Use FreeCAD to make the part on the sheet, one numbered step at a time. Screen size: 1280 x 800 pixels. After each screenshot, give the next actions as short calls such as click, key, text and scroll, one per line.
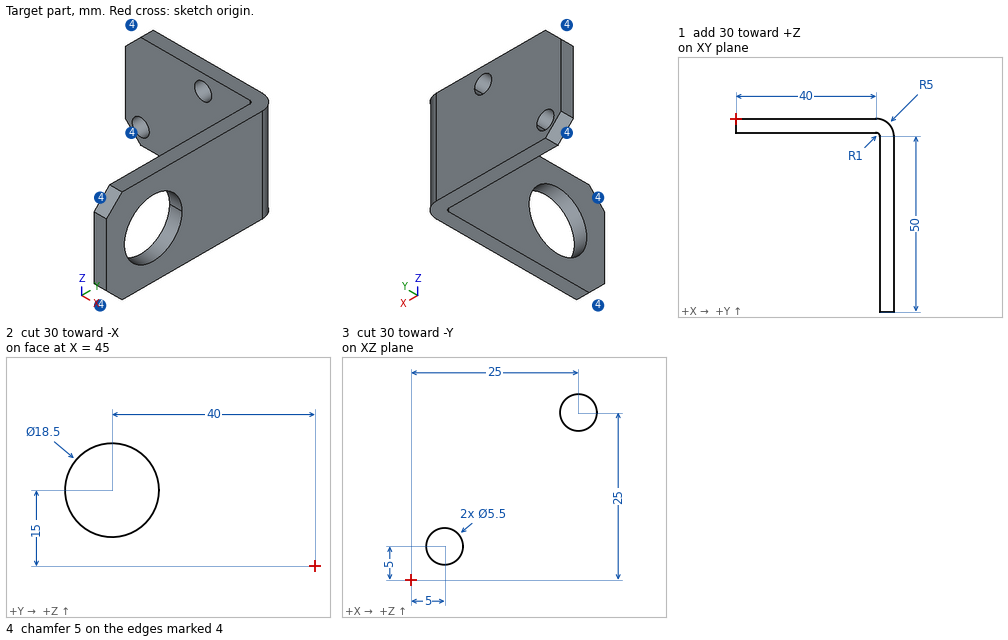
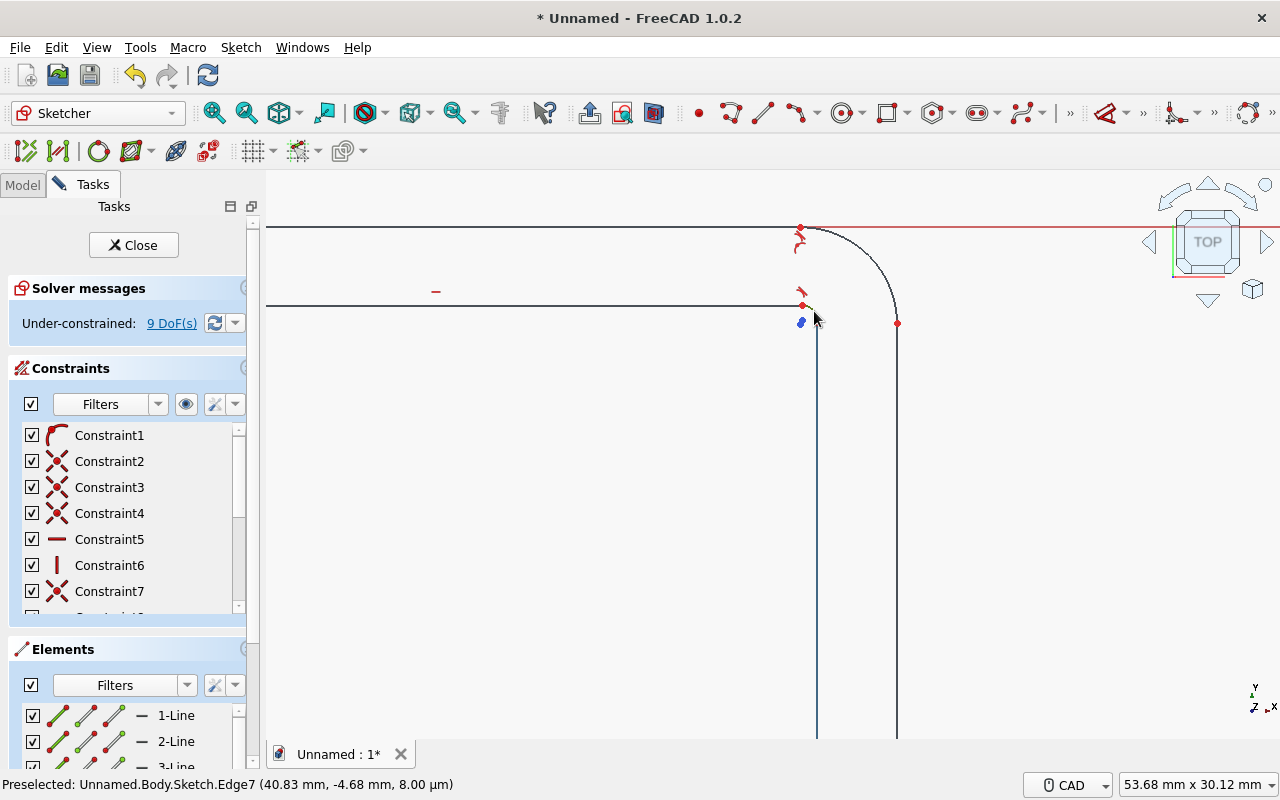
key(t)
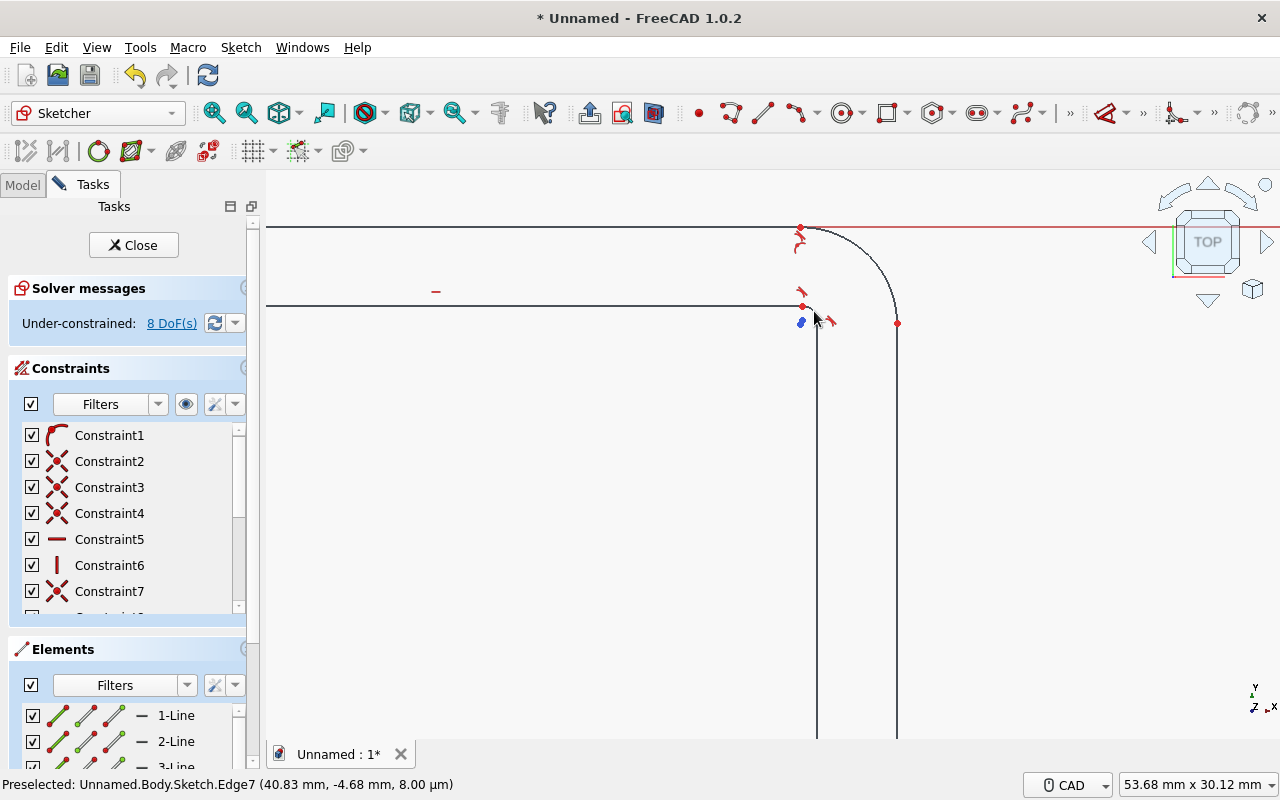
click(897, 608)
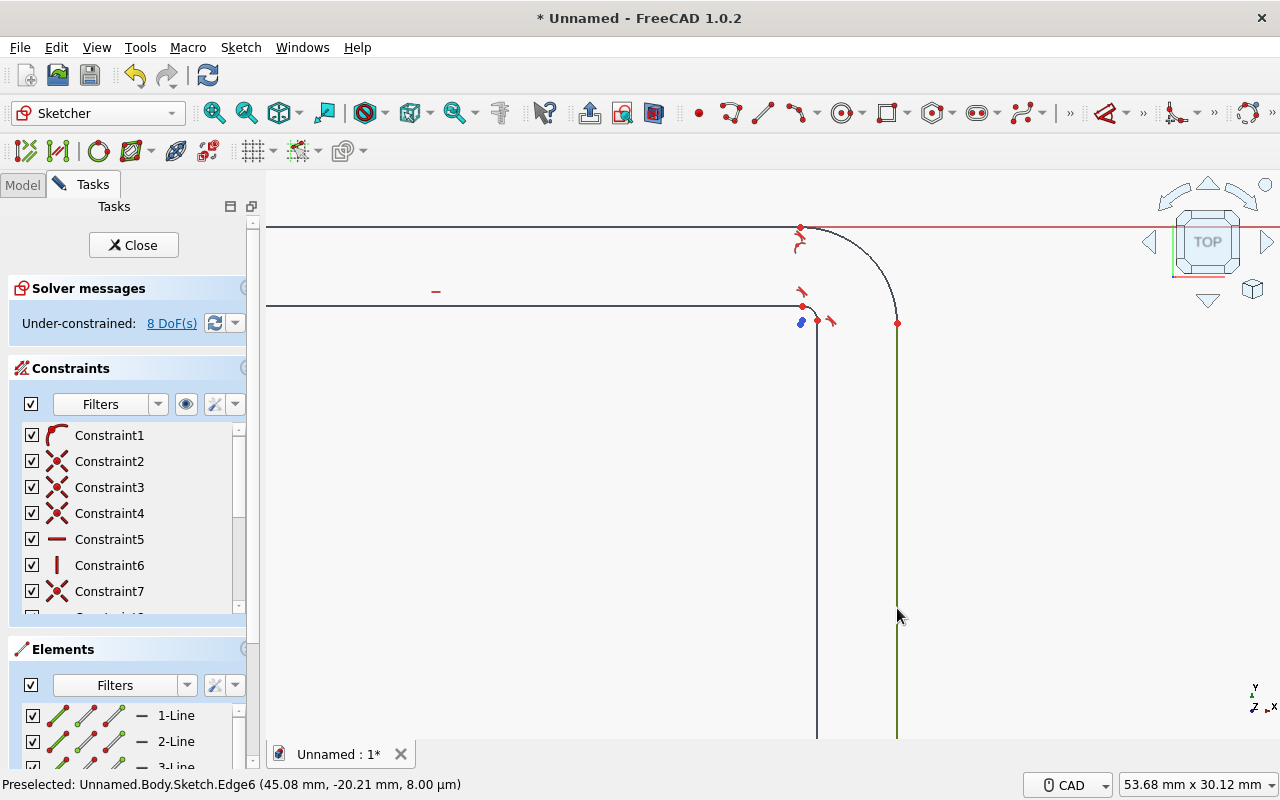
click(886, 280)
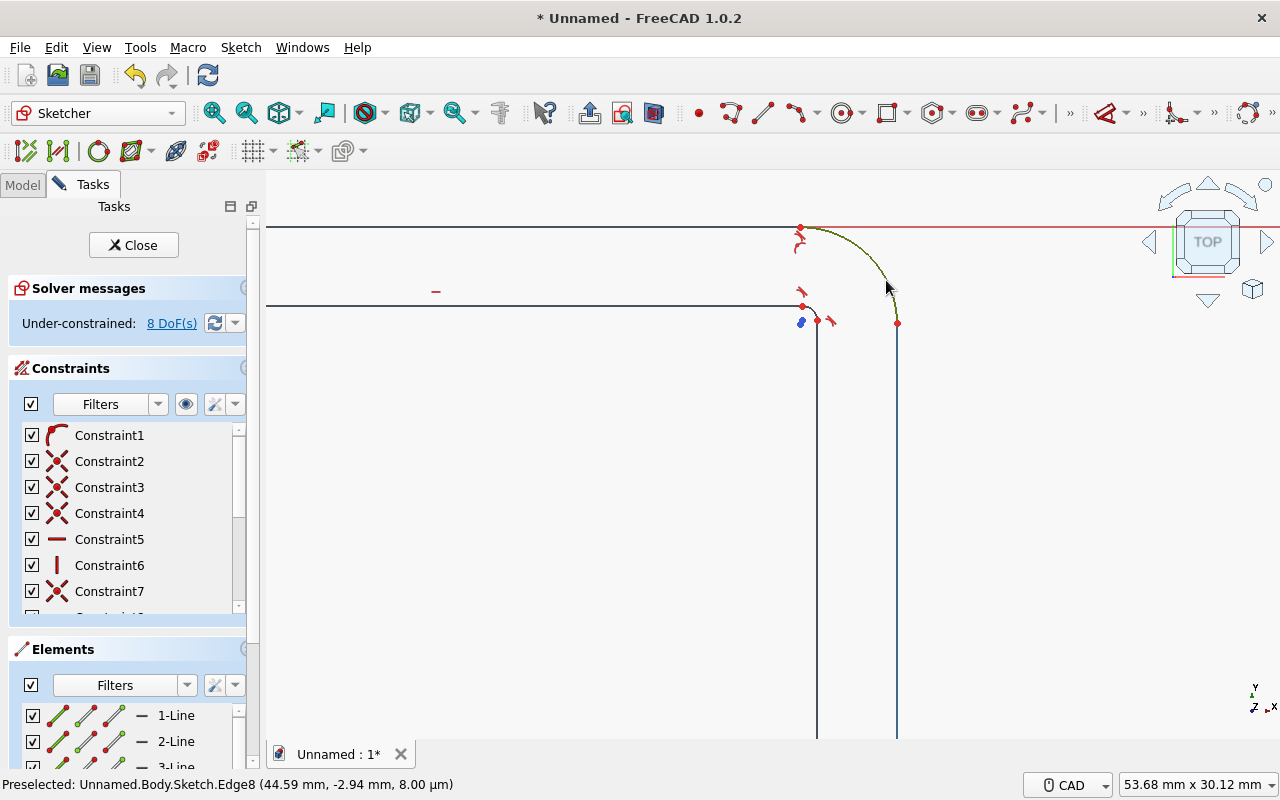
key(t)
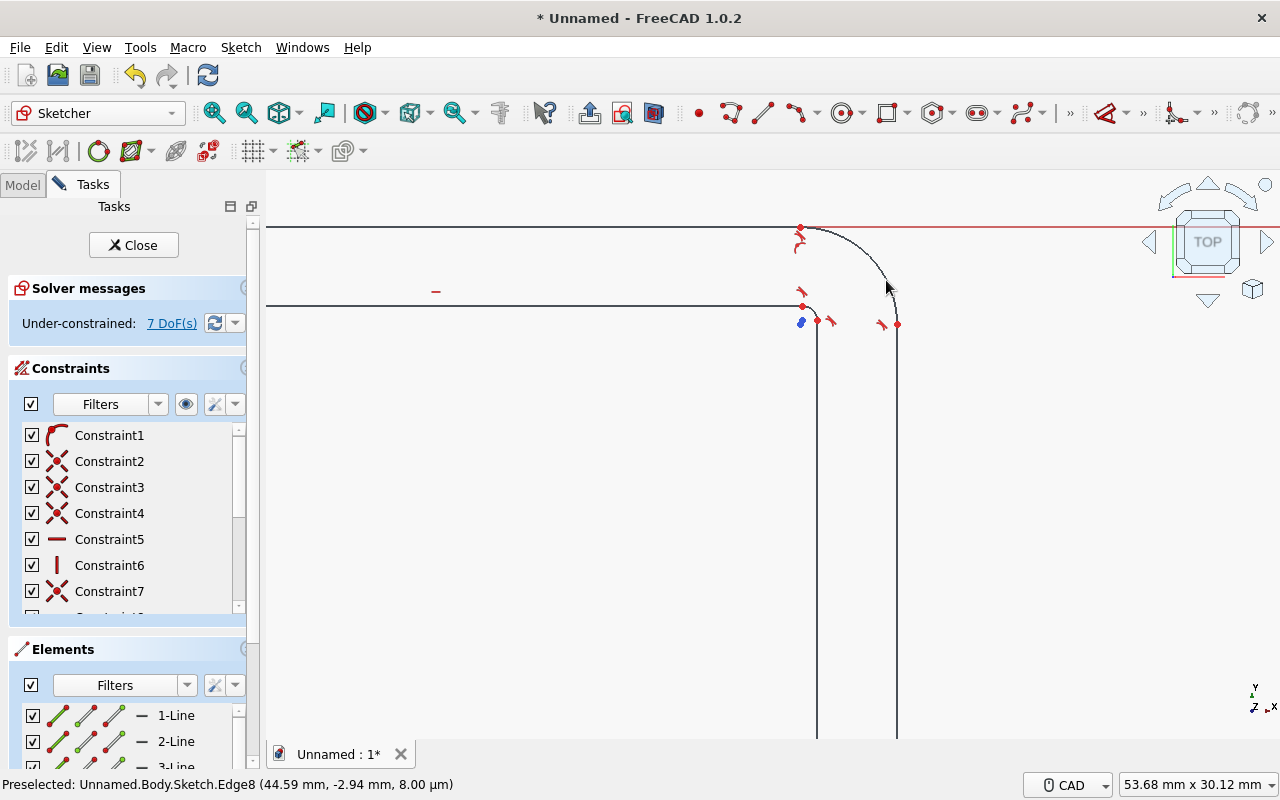
scroll(841, 284, down, 5)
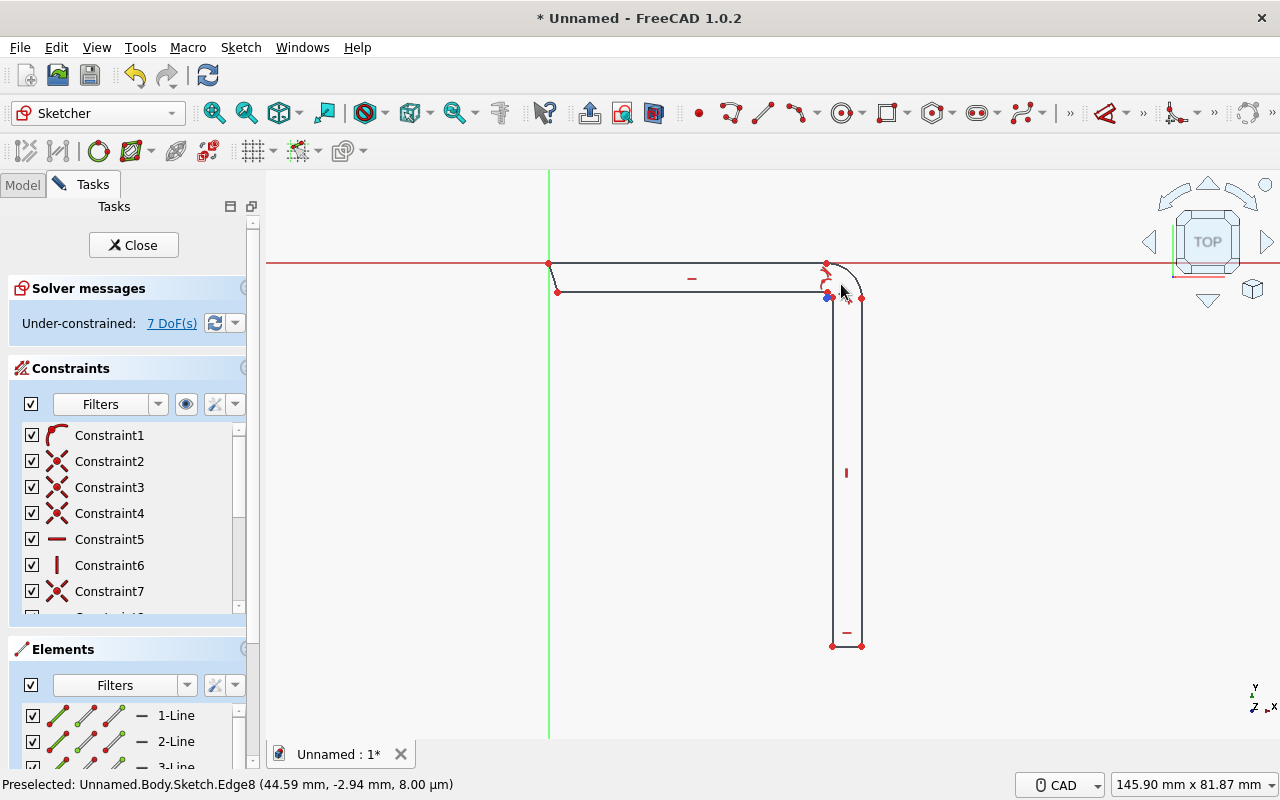
scroll(555, 284, up, 4)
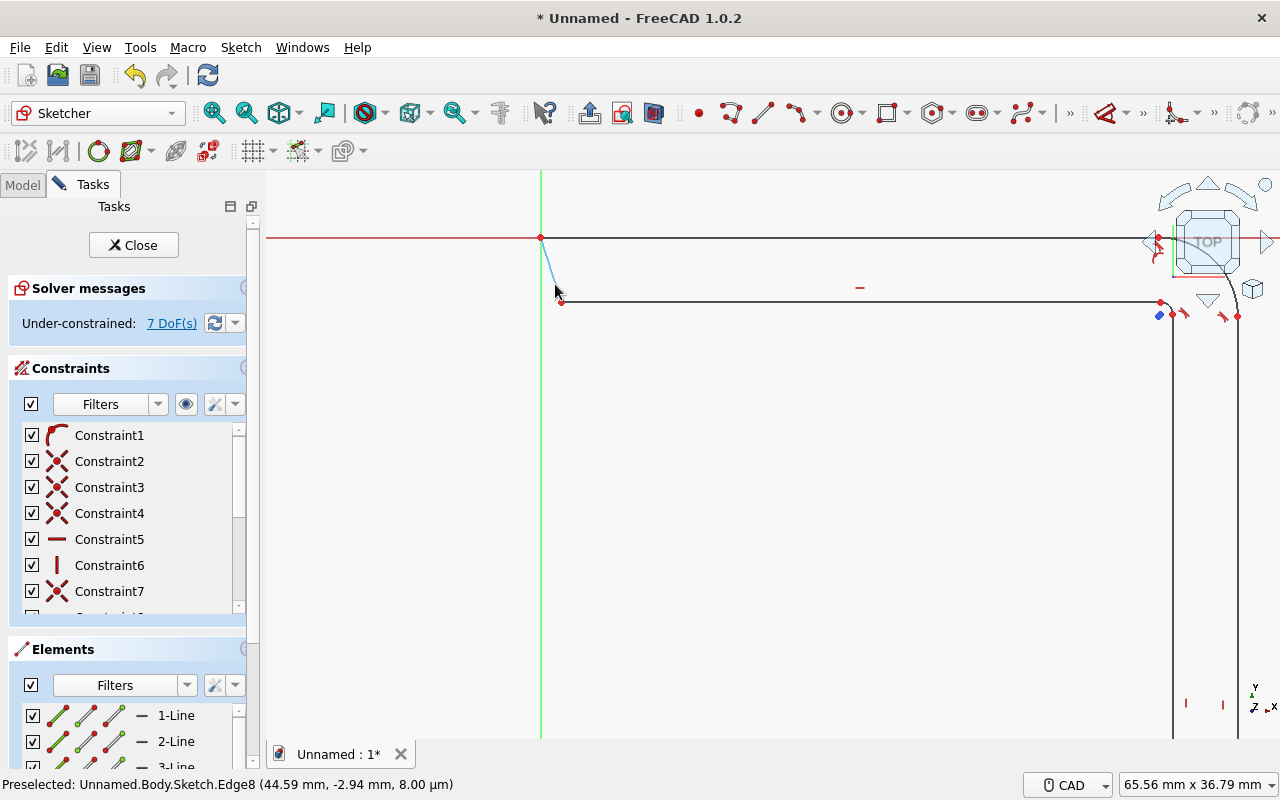
click(555, 283)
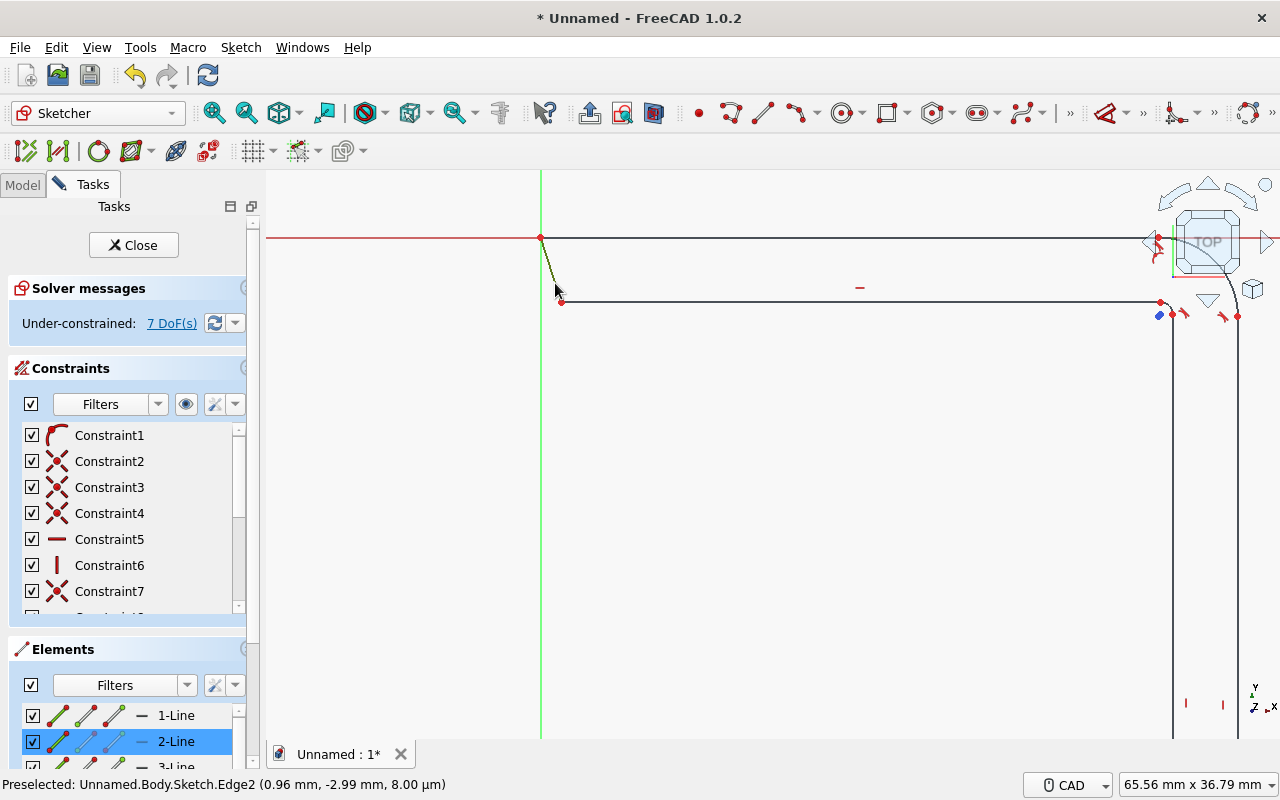
key(v)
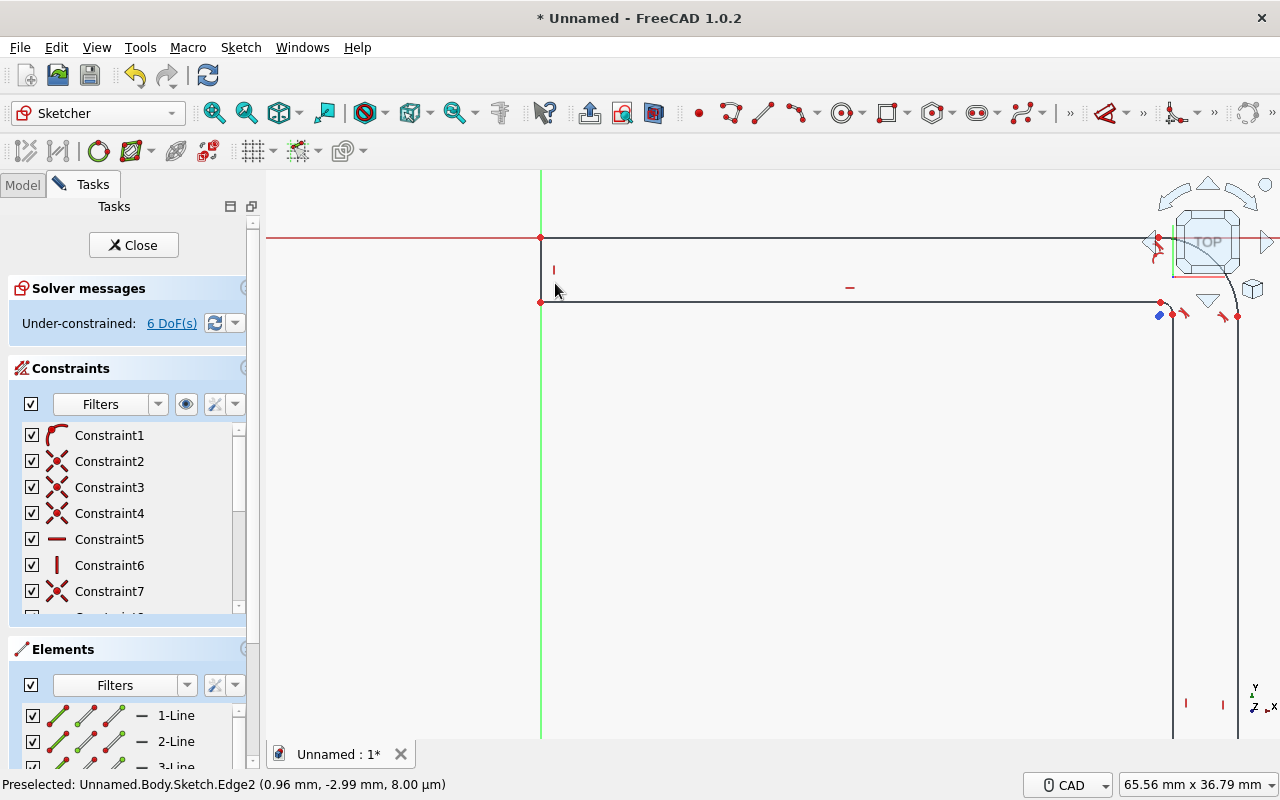
scroll(554, 284, down, 4)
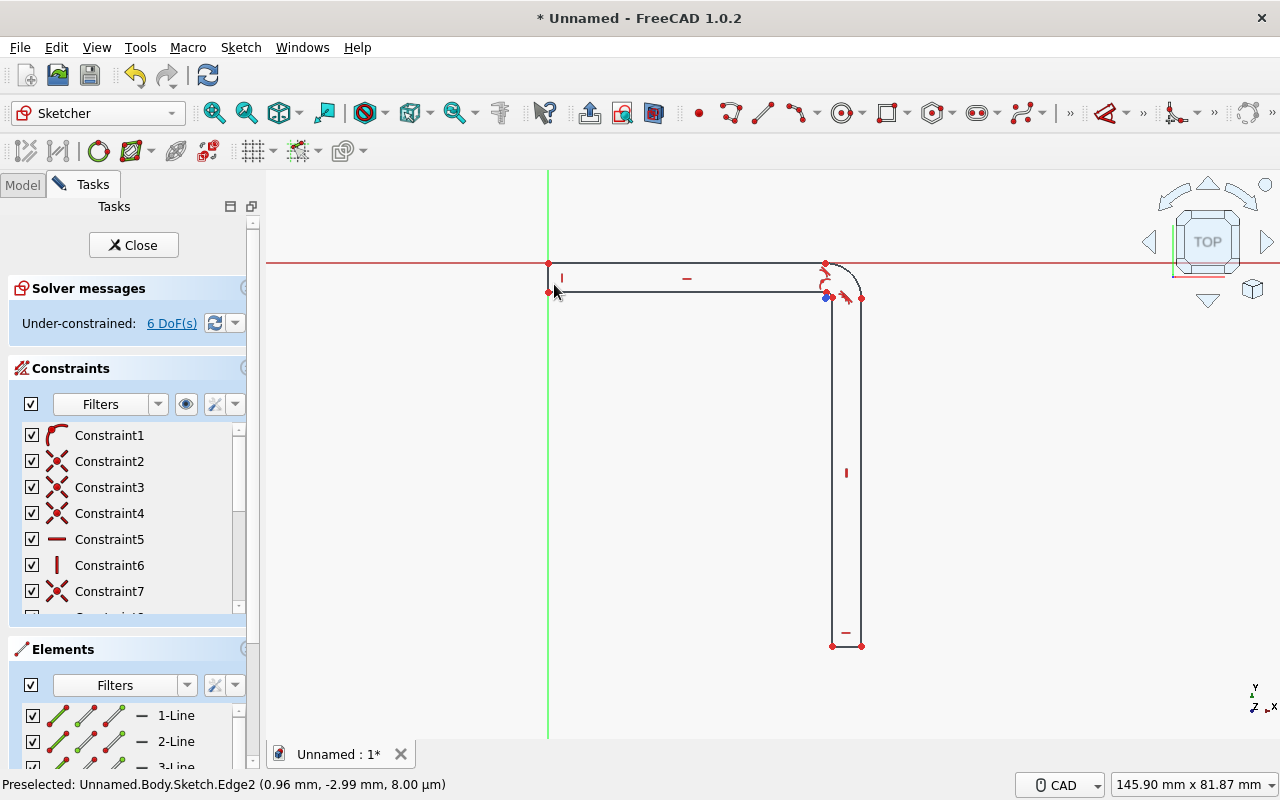
scroll(831, 294, up, 7)